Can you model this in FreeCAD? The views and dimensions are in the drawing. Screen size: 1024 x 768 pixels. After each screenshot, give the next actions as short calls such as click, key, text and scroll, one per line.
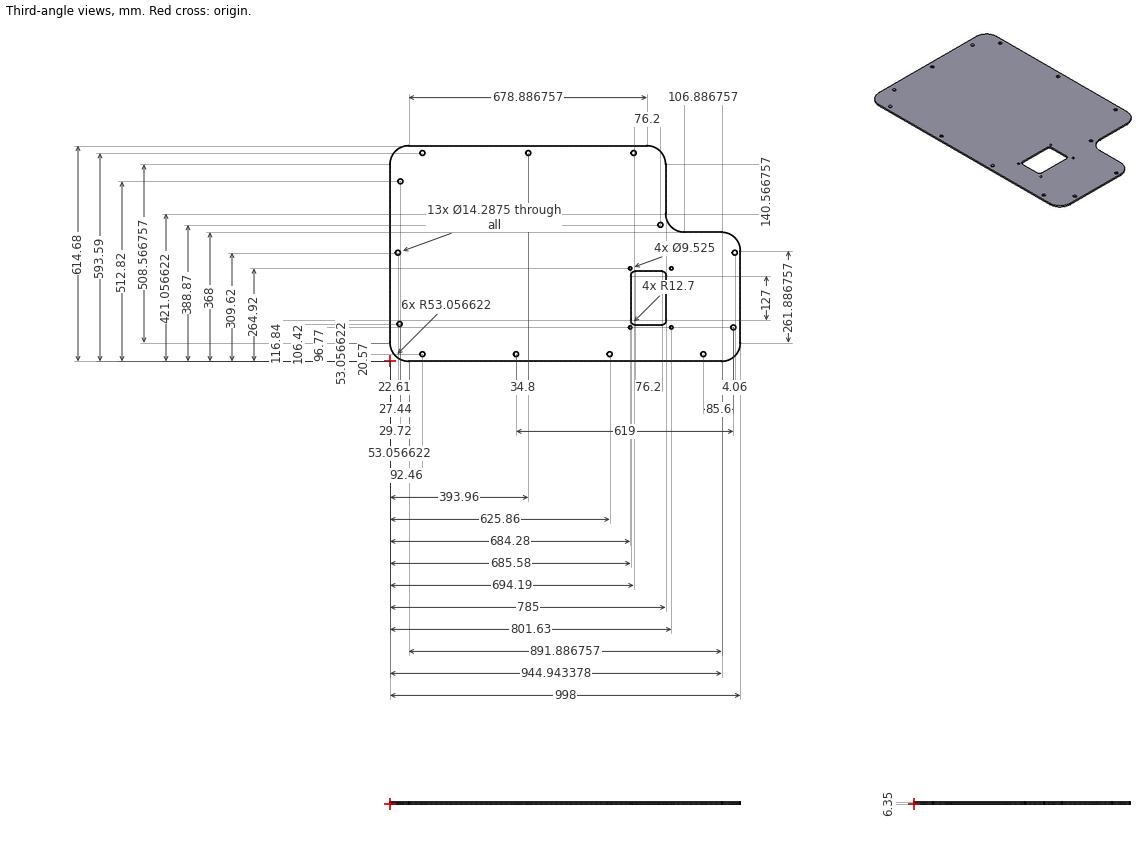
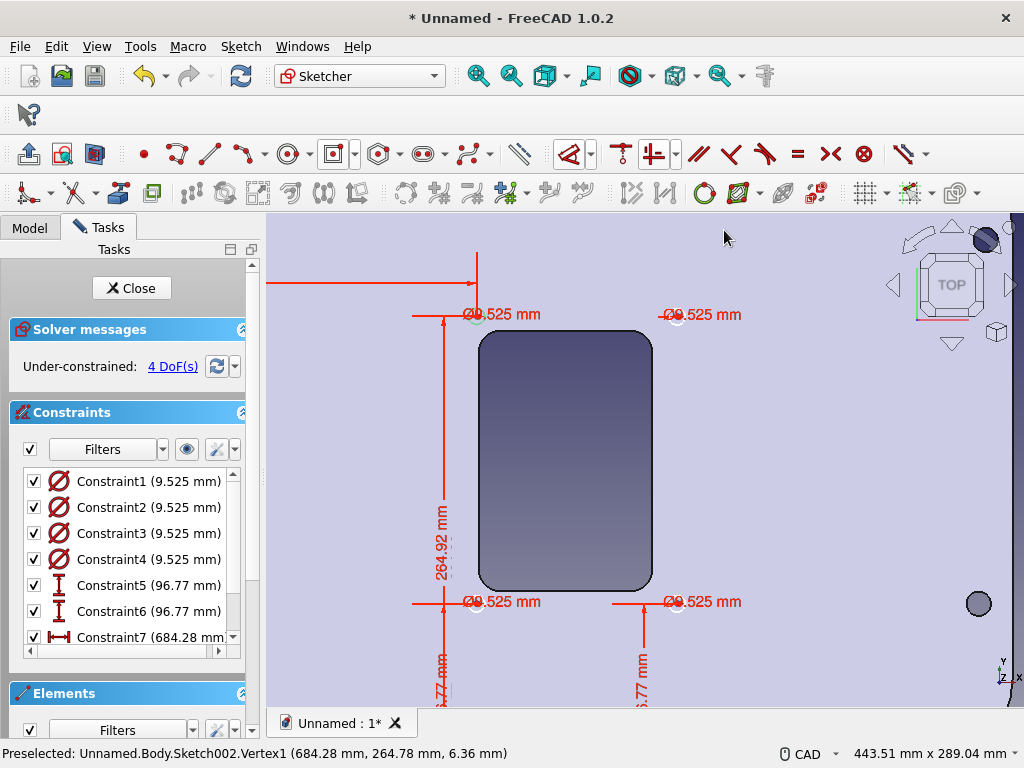
click(477, 604)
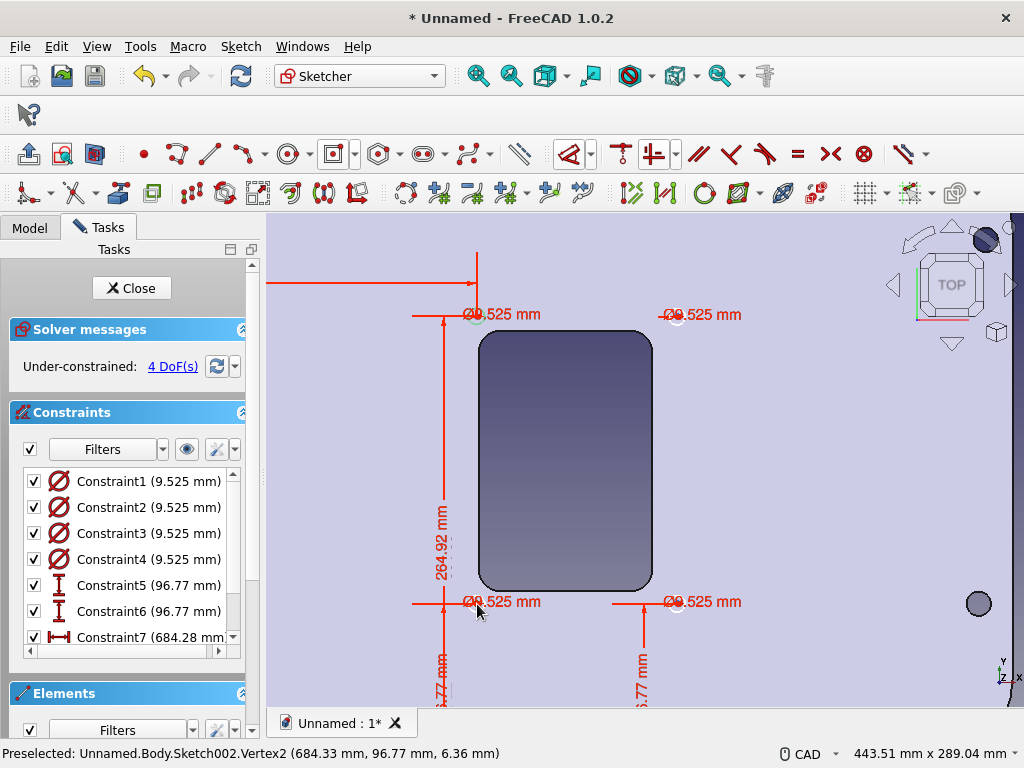
click(590, 154)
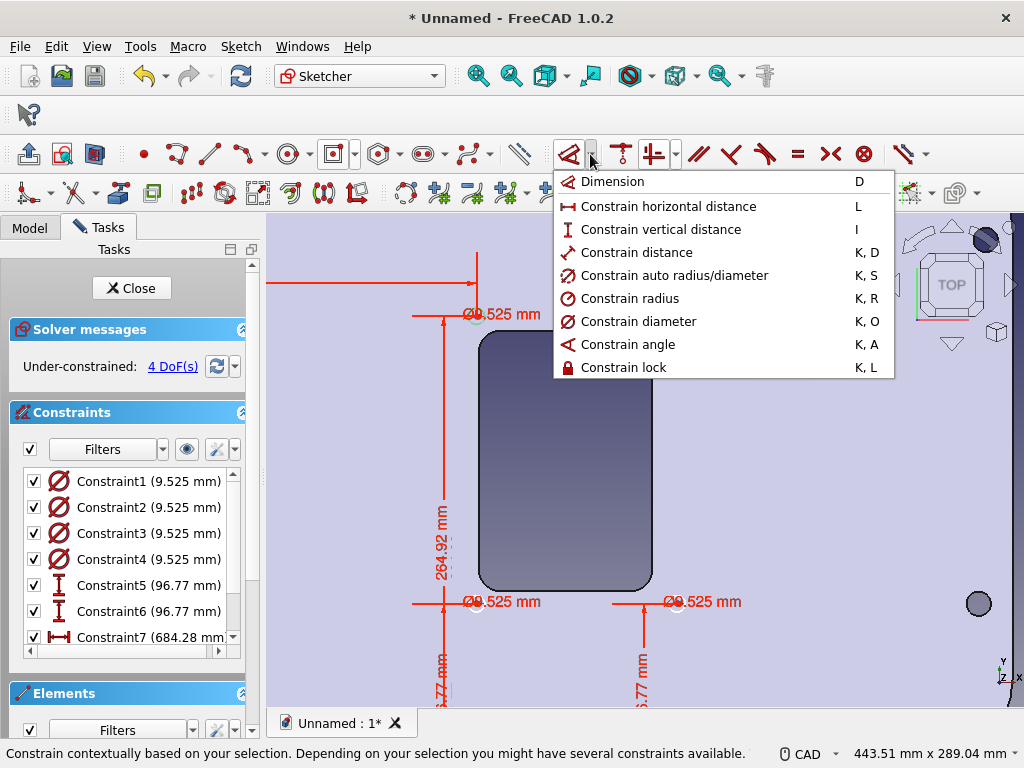
click(724, 206)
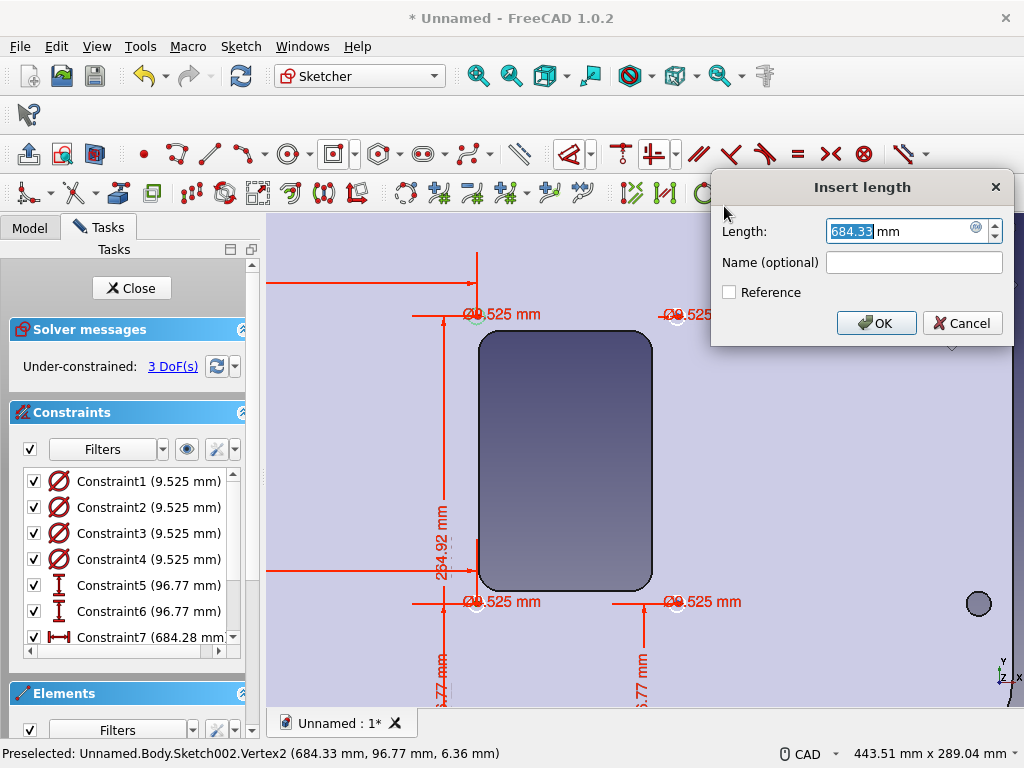
text(684.28)
key(Return)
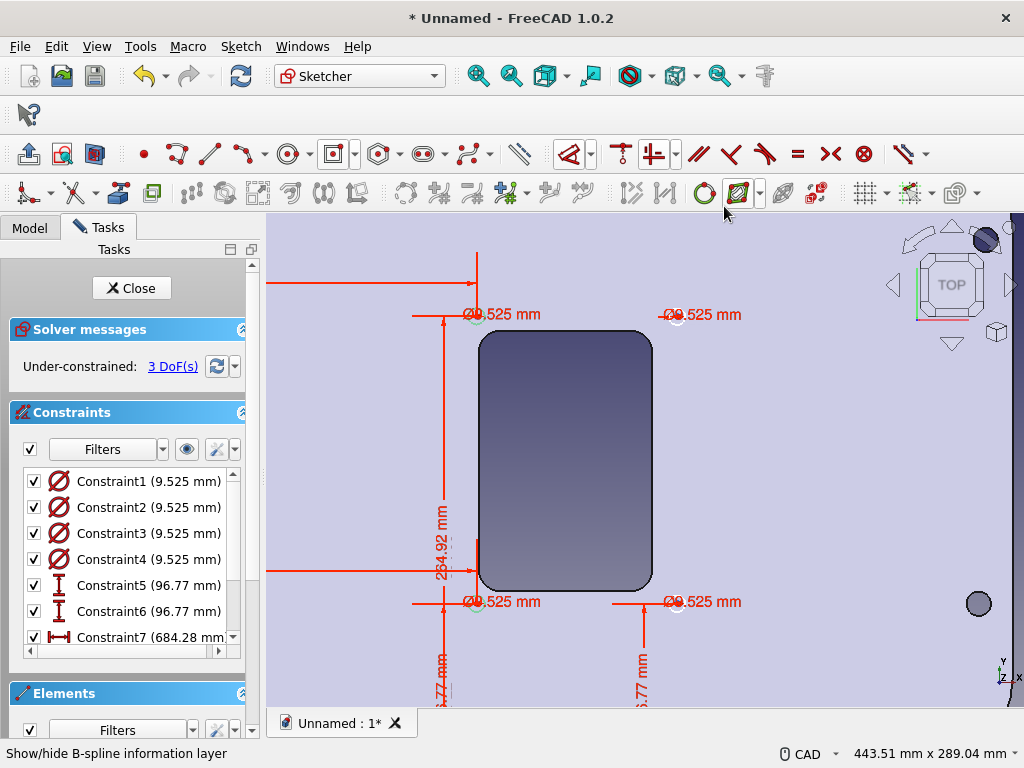
click(677, 604)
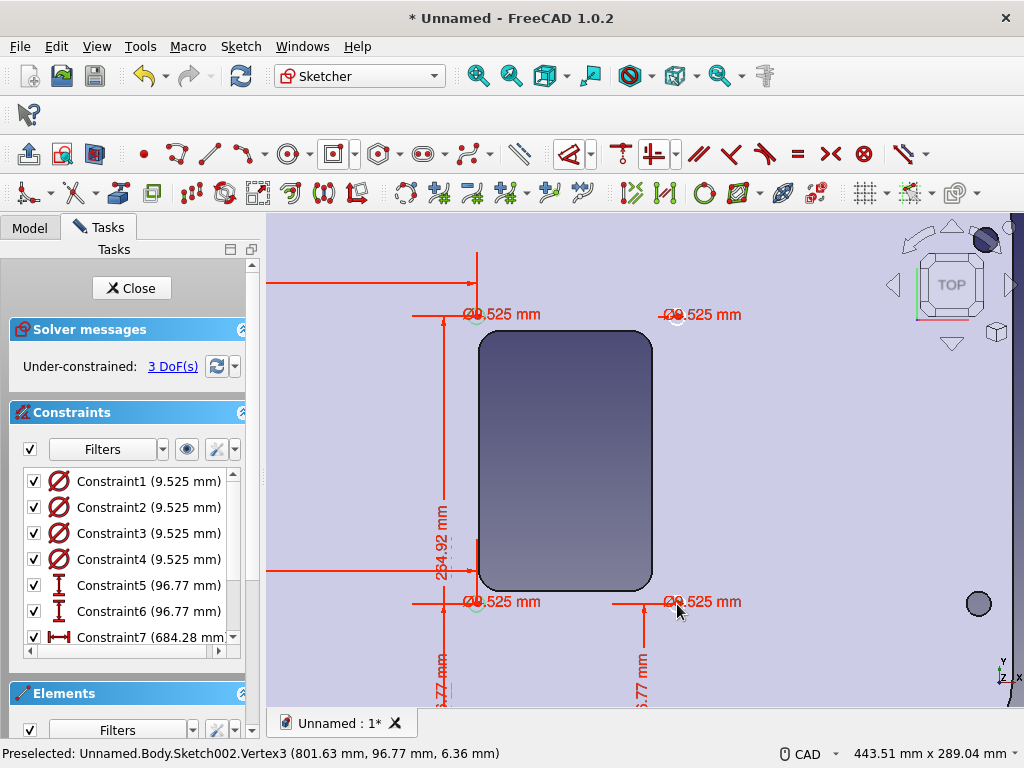
click(590, 154)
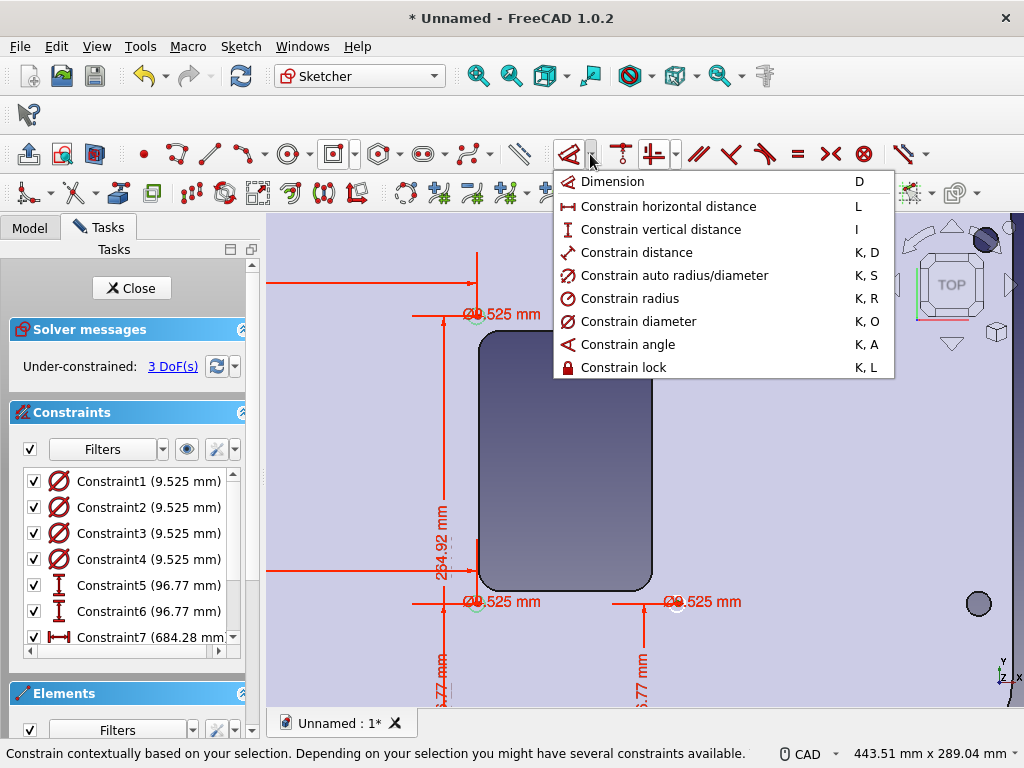
click(724, 206)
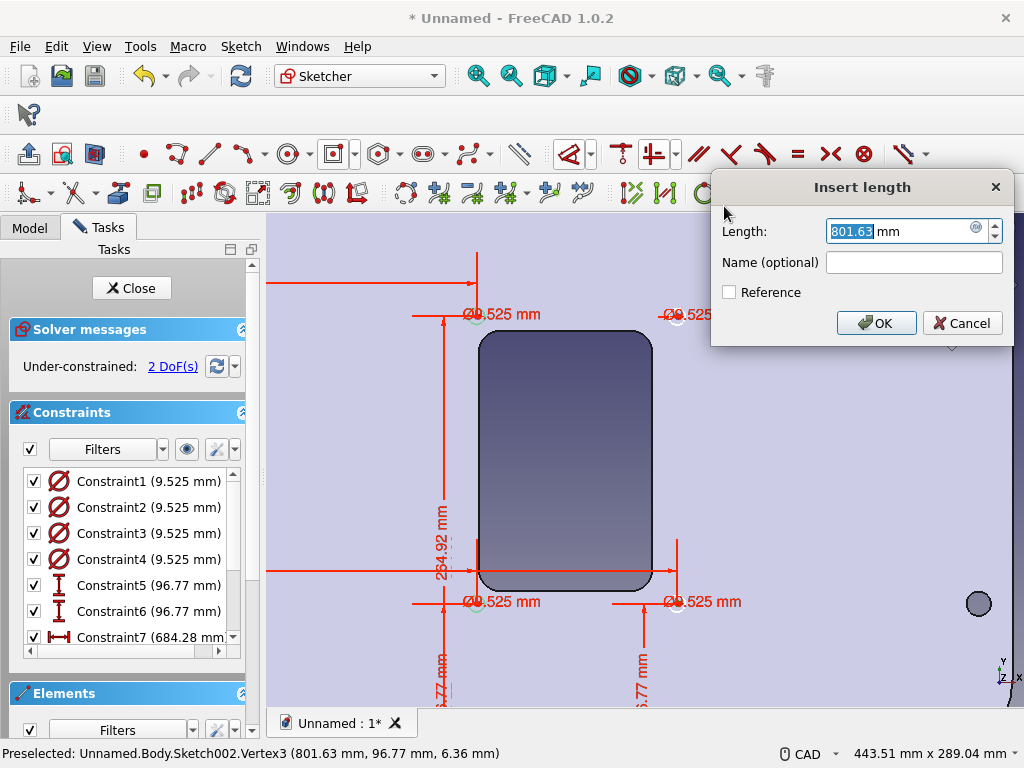
text(801.63)
key(Return)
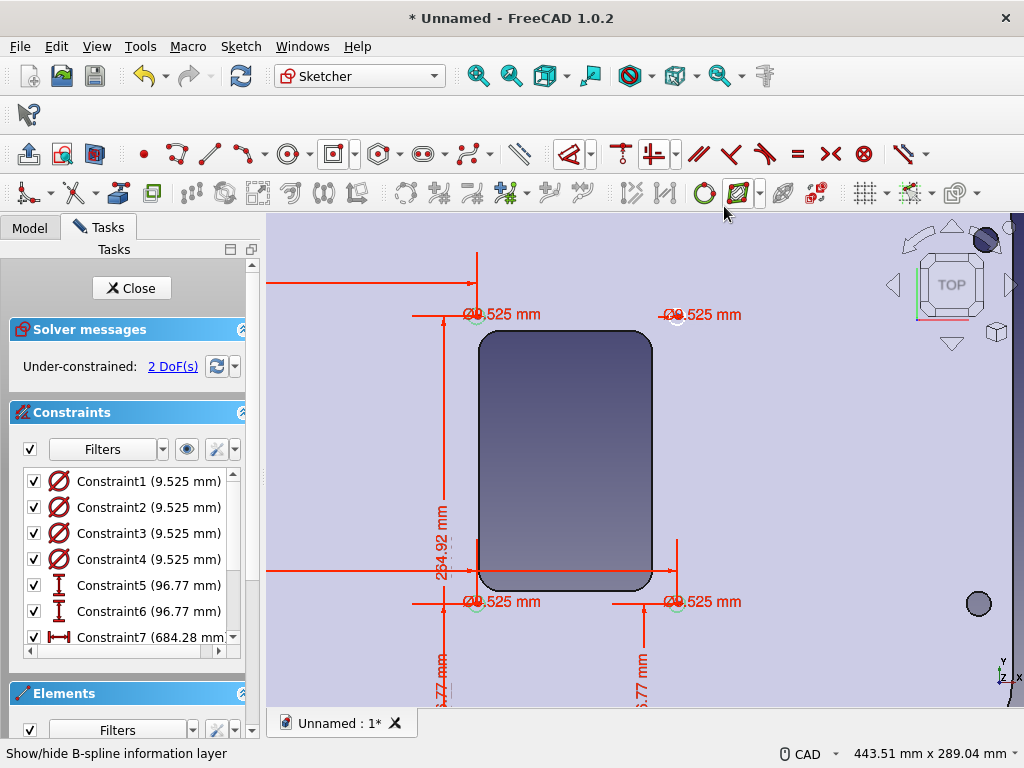
click(677, 317)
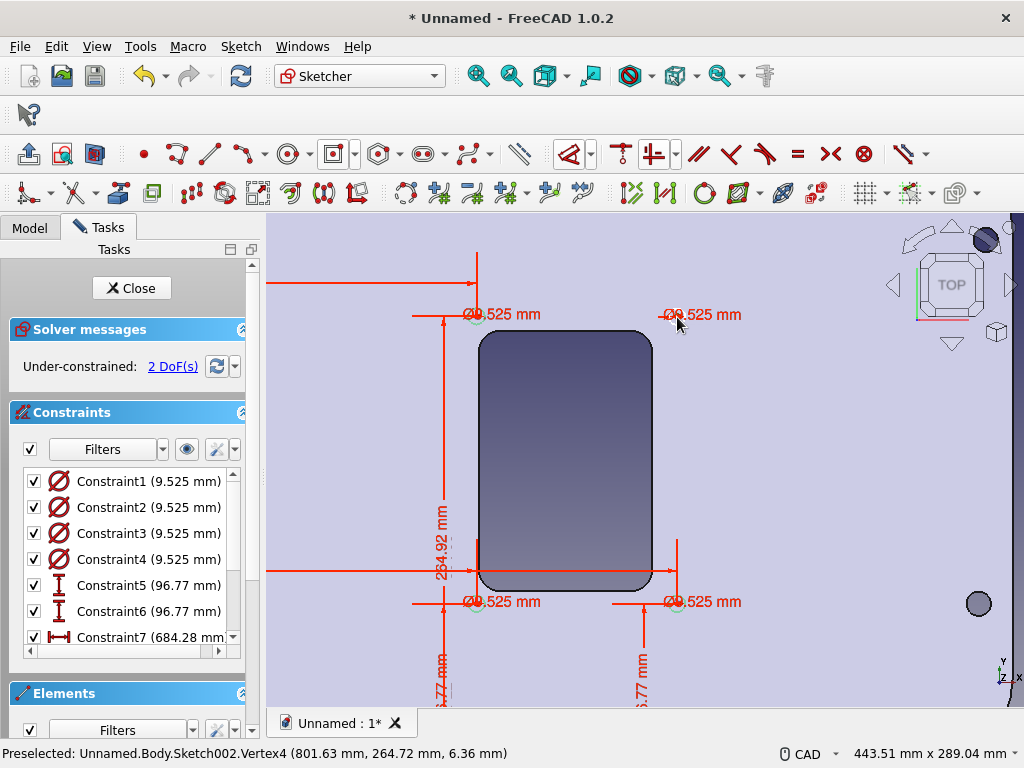
key(l)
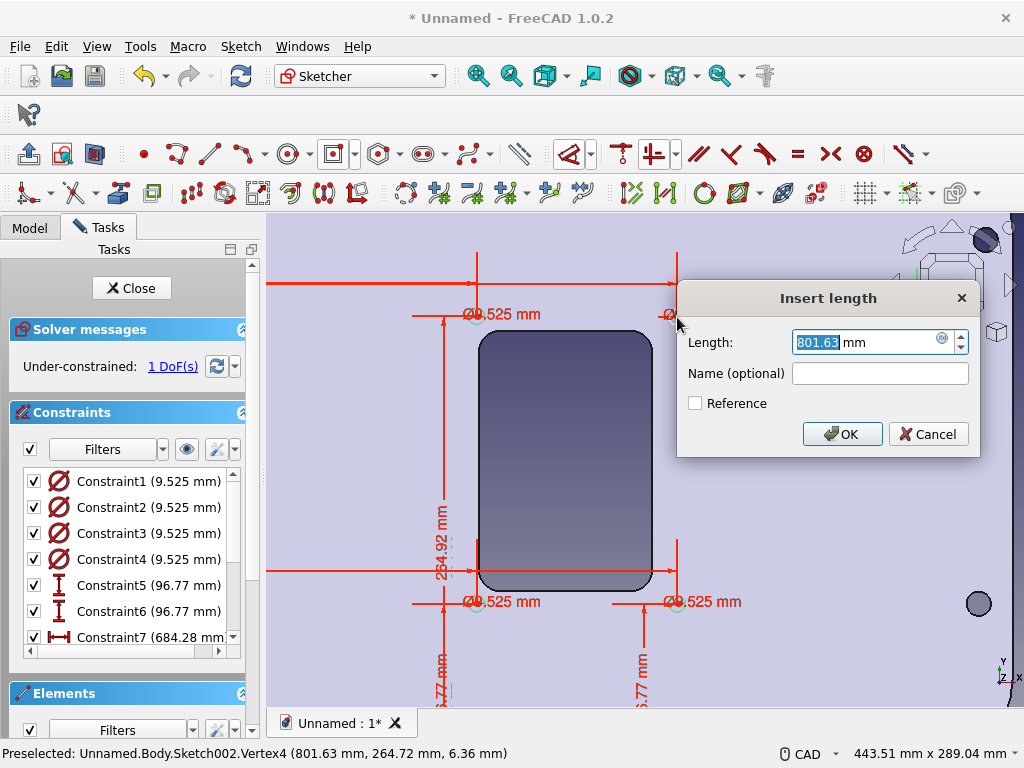
text(801.63)
key(Return)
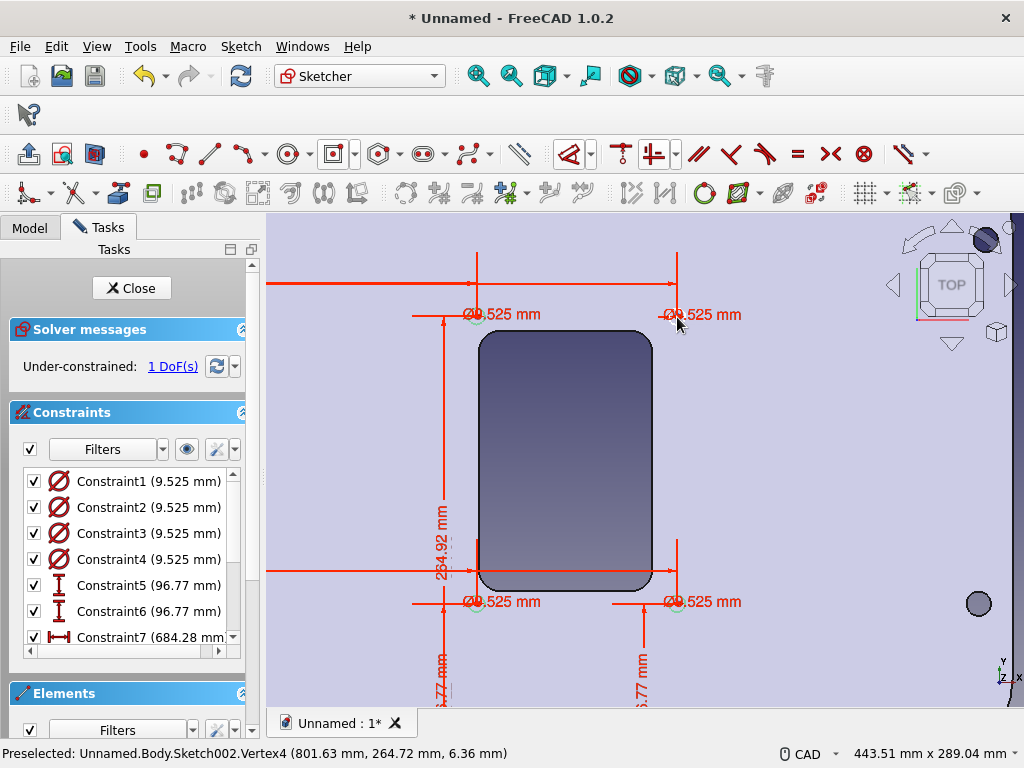
click(677, 317)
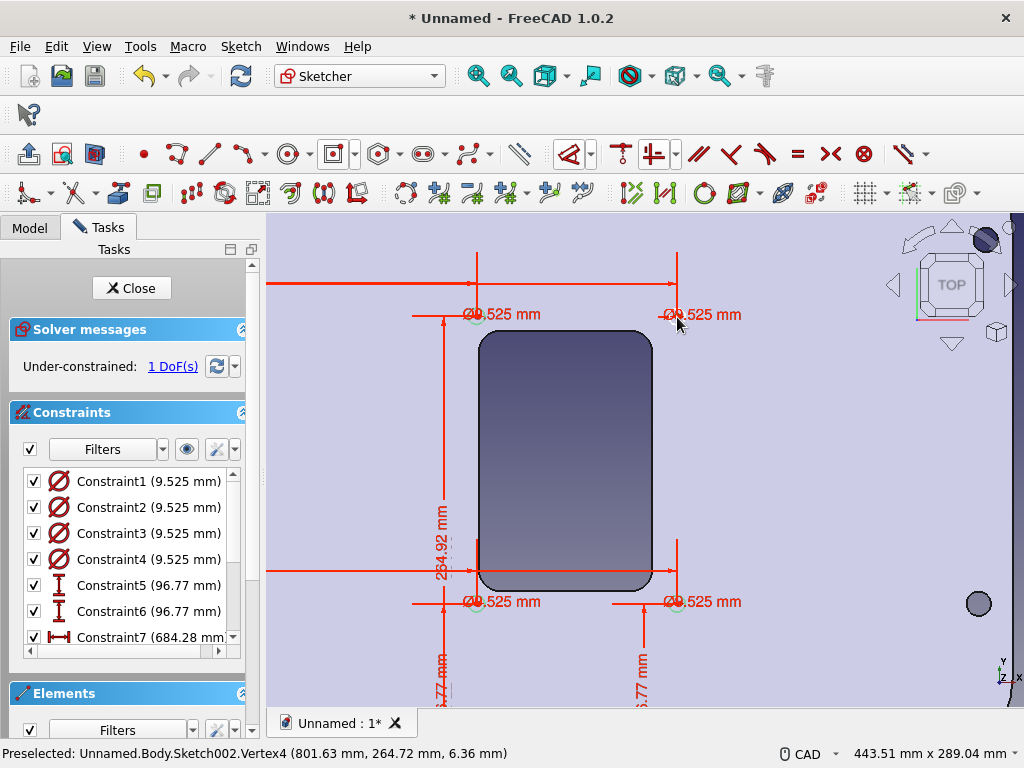
key(i)